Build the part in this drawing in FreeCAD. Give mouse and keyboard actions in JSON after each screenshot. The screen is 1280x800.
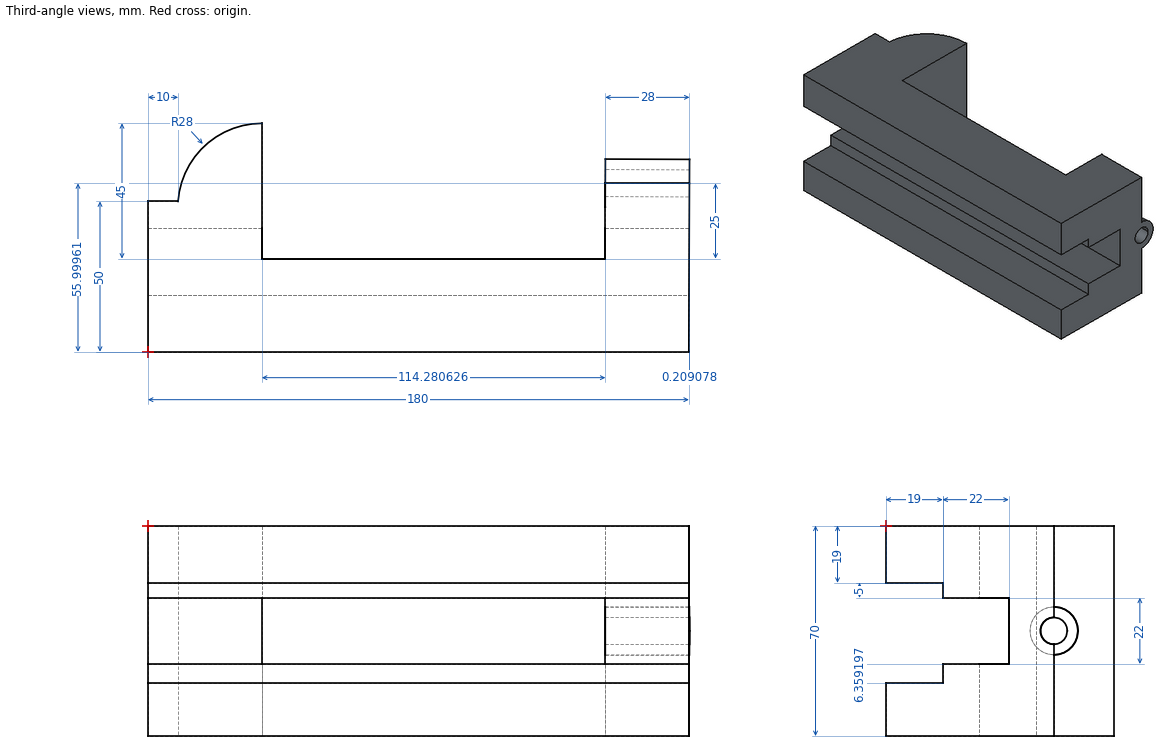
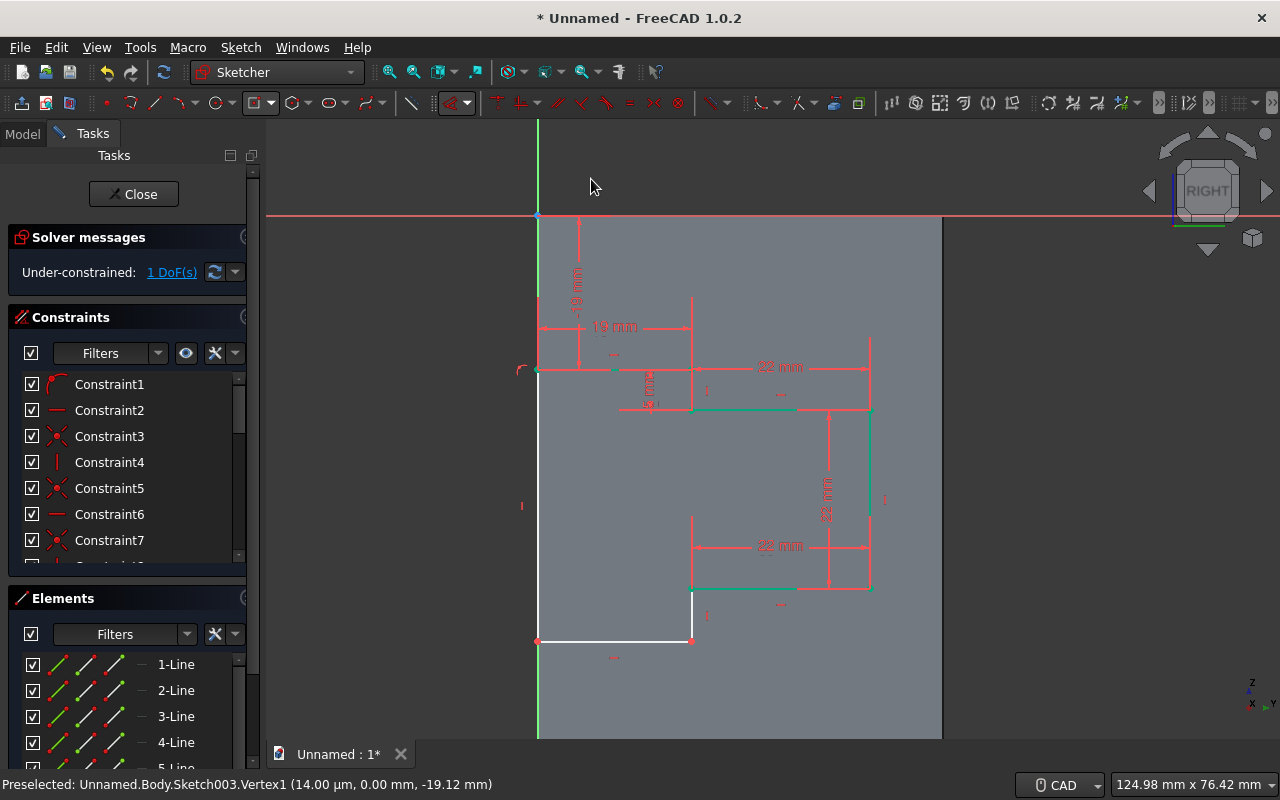
{"action": "left_click", "coordinate": [692, 605]}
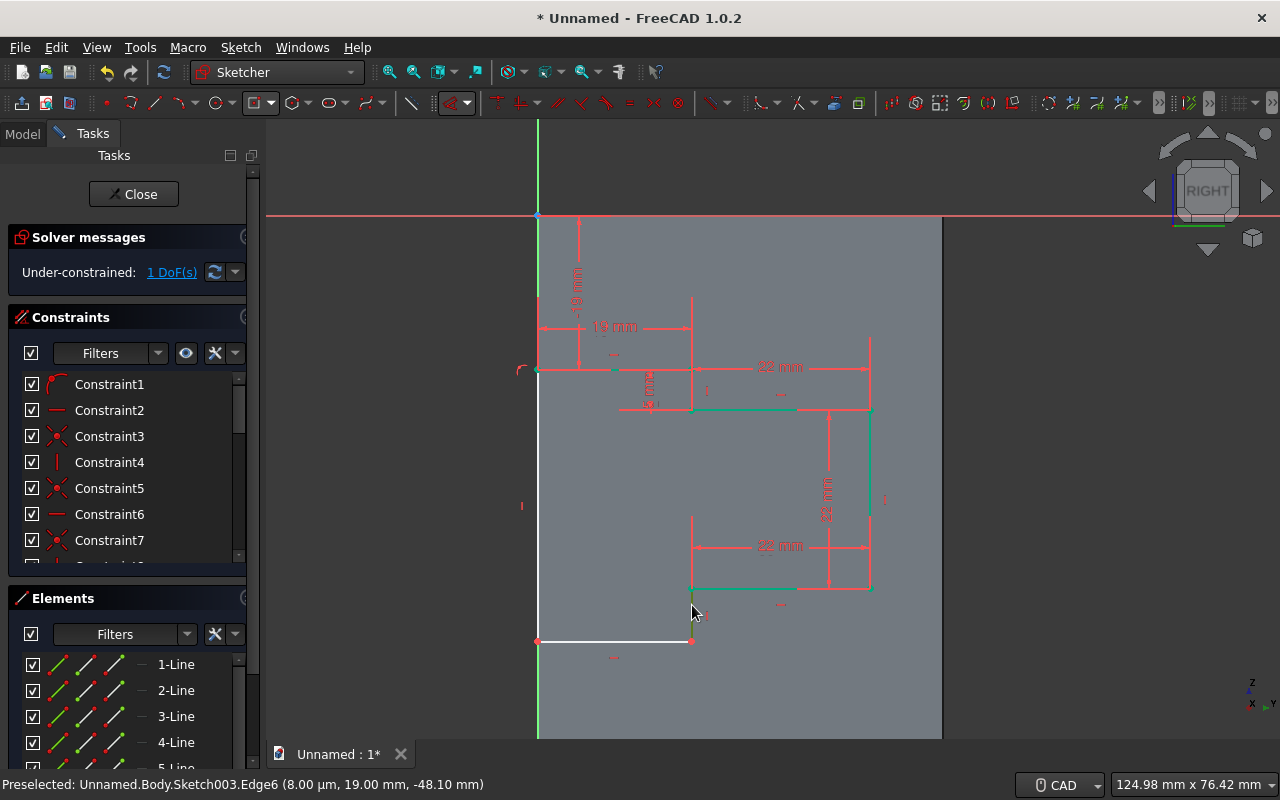
{"action": "left_click", "coordinate": [470, 104]}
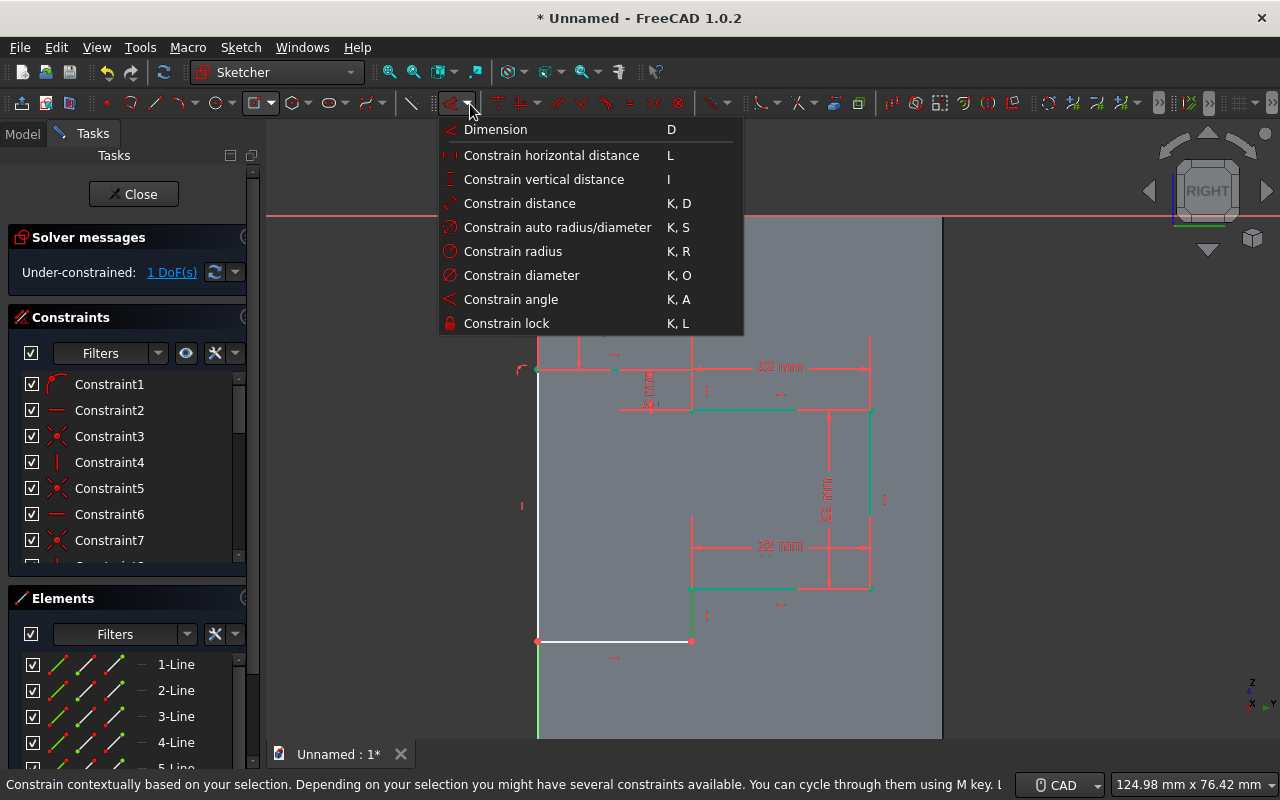
{"action": "left_click", "coordinate": [591, 179]}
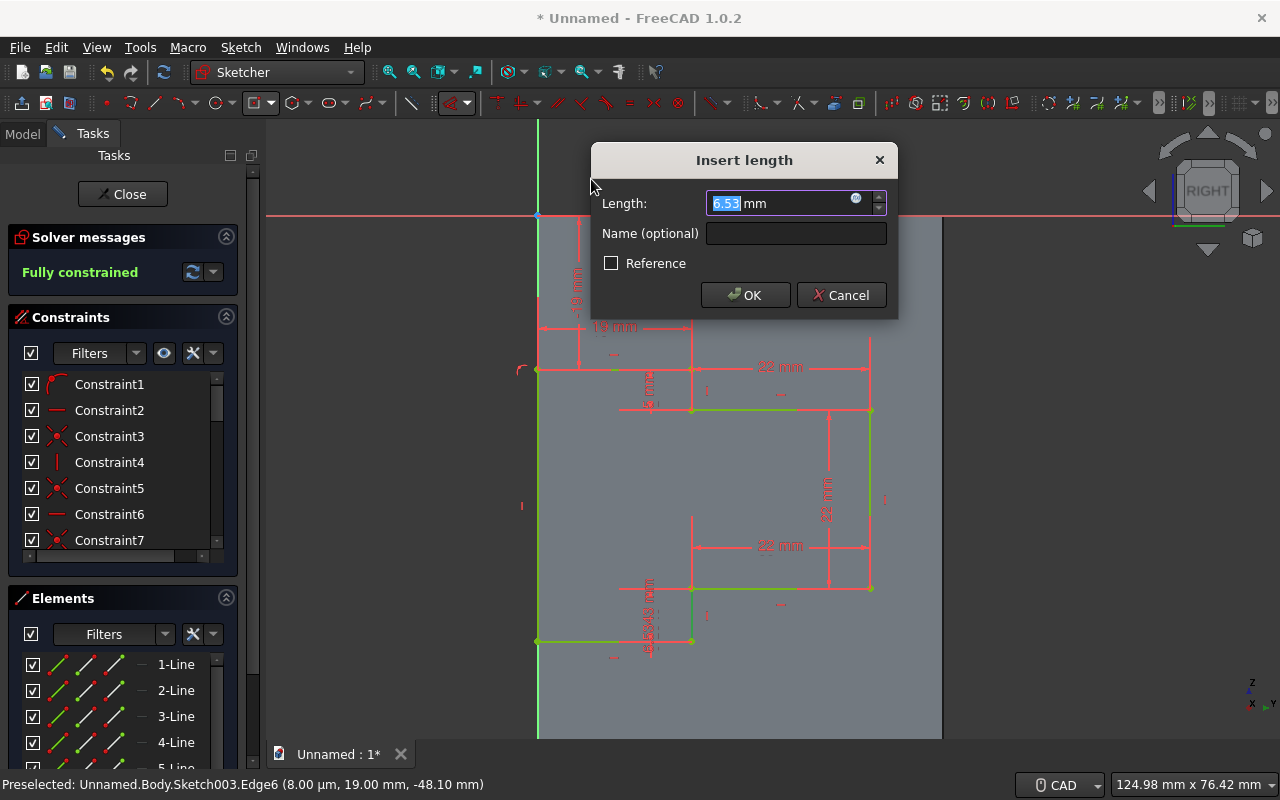
{"action": "type", "text": "6.359197"}
{"action": "key", "text": "Return"}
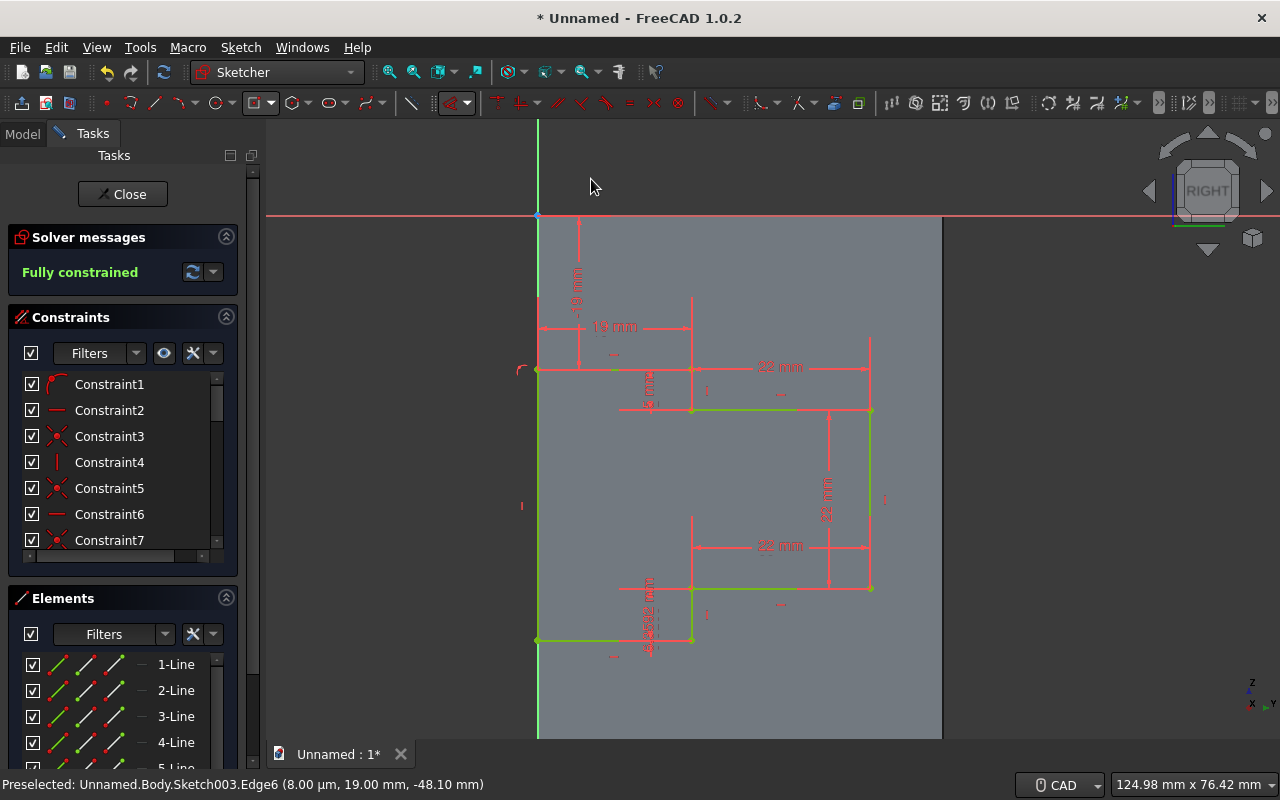
{"action": "left_click", "coordinate": [123, 194]}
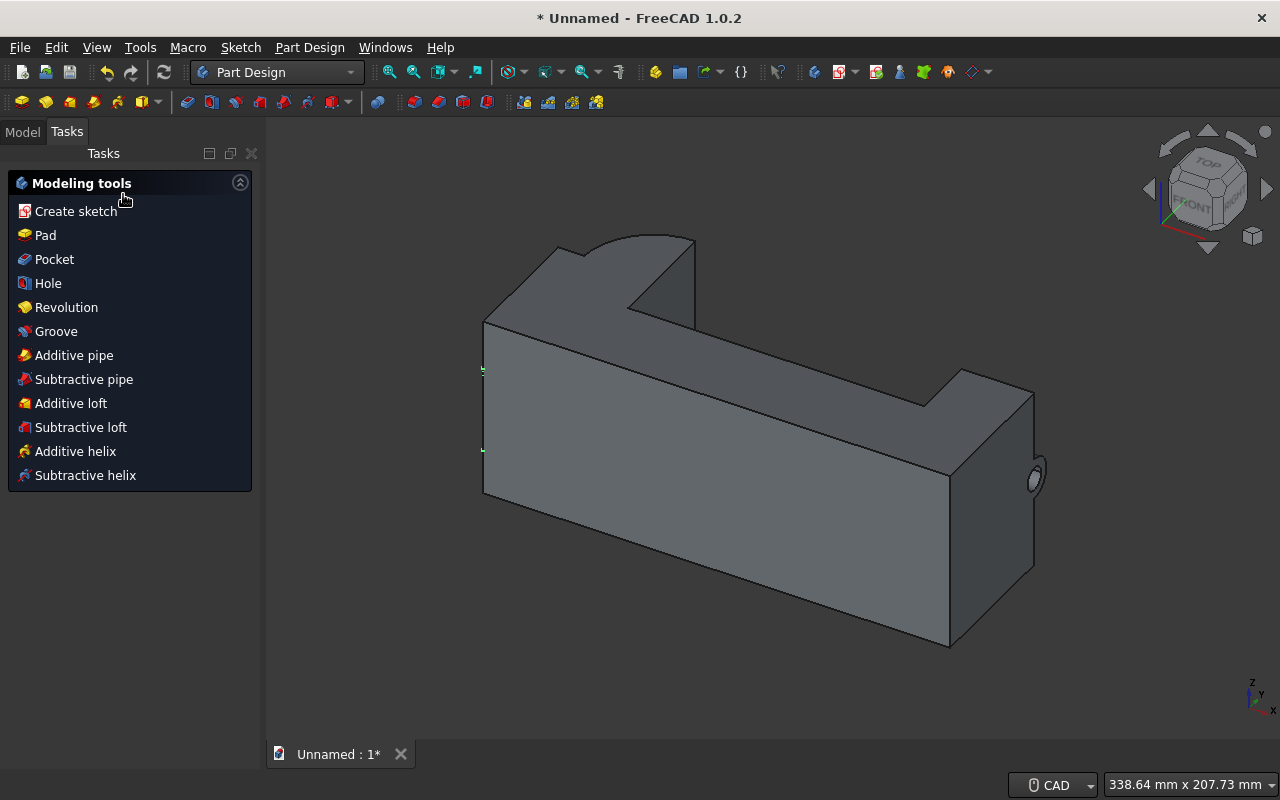
{"action": "left_click", "coordinate": [188, 102]}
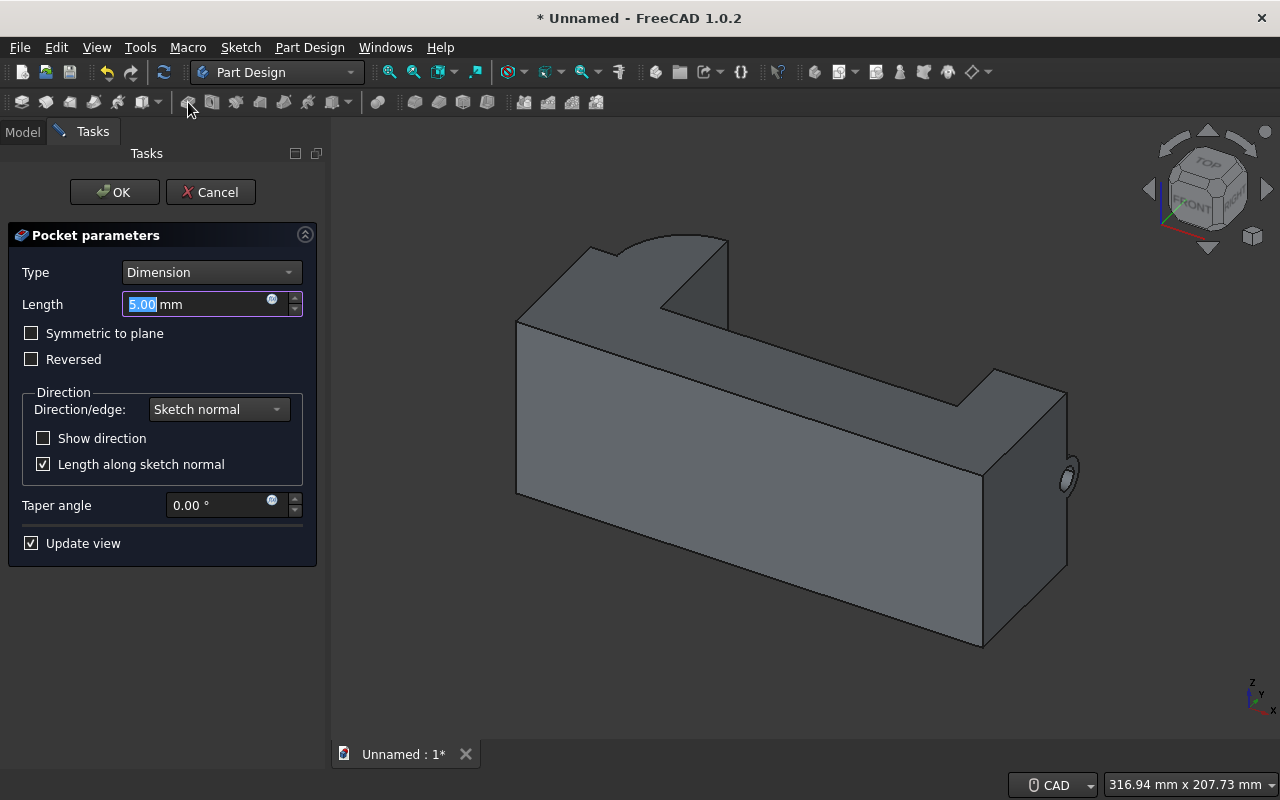
{"action": "left_click", "coordinate": [212, 272]}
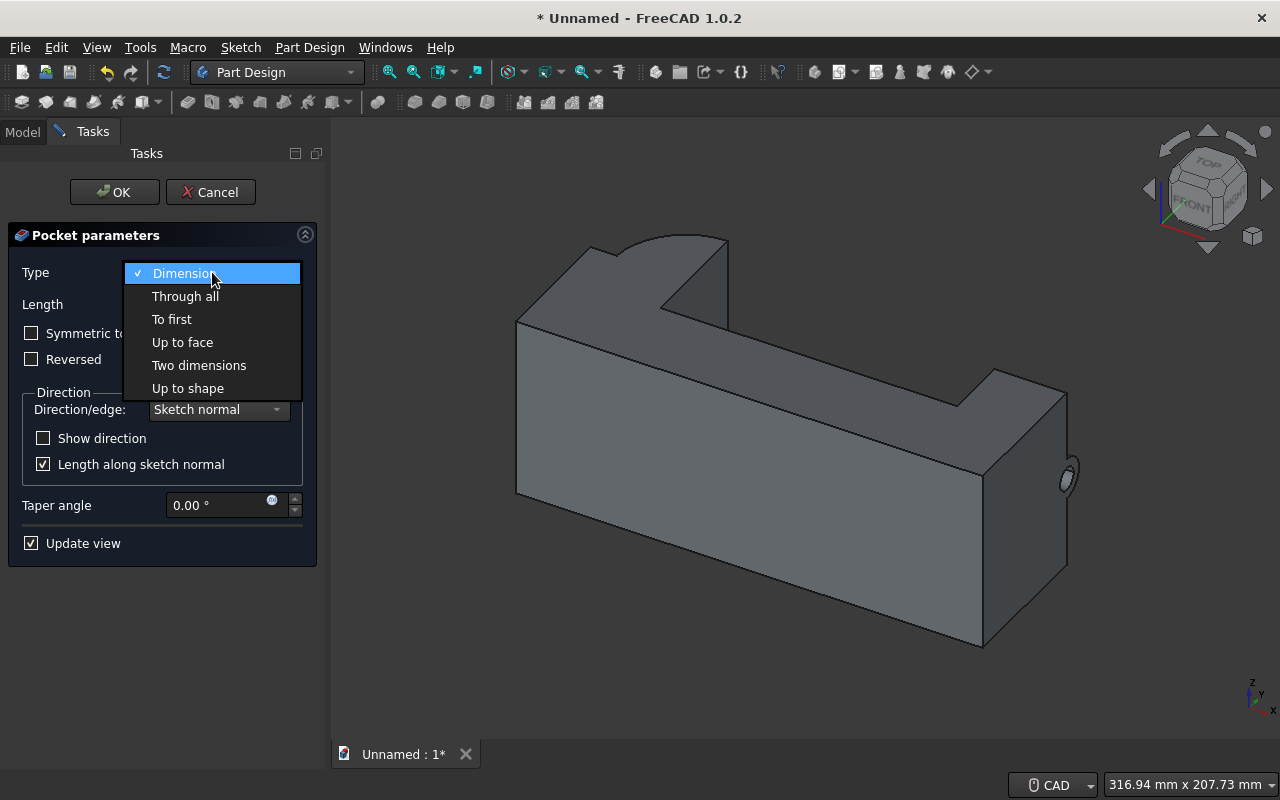
{"action": "left_click", "coordinate": [212, 296]}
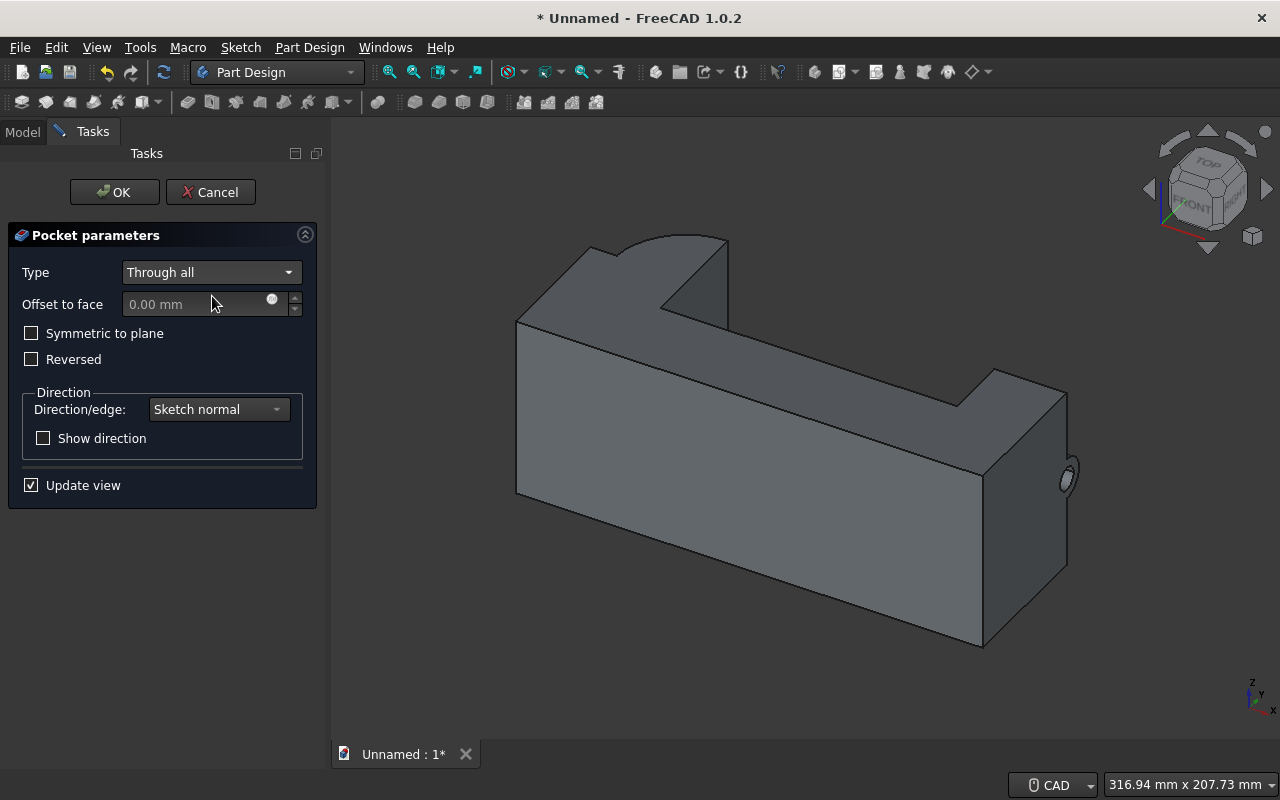
{"action": "left_click", "coordinate": [30, 359]}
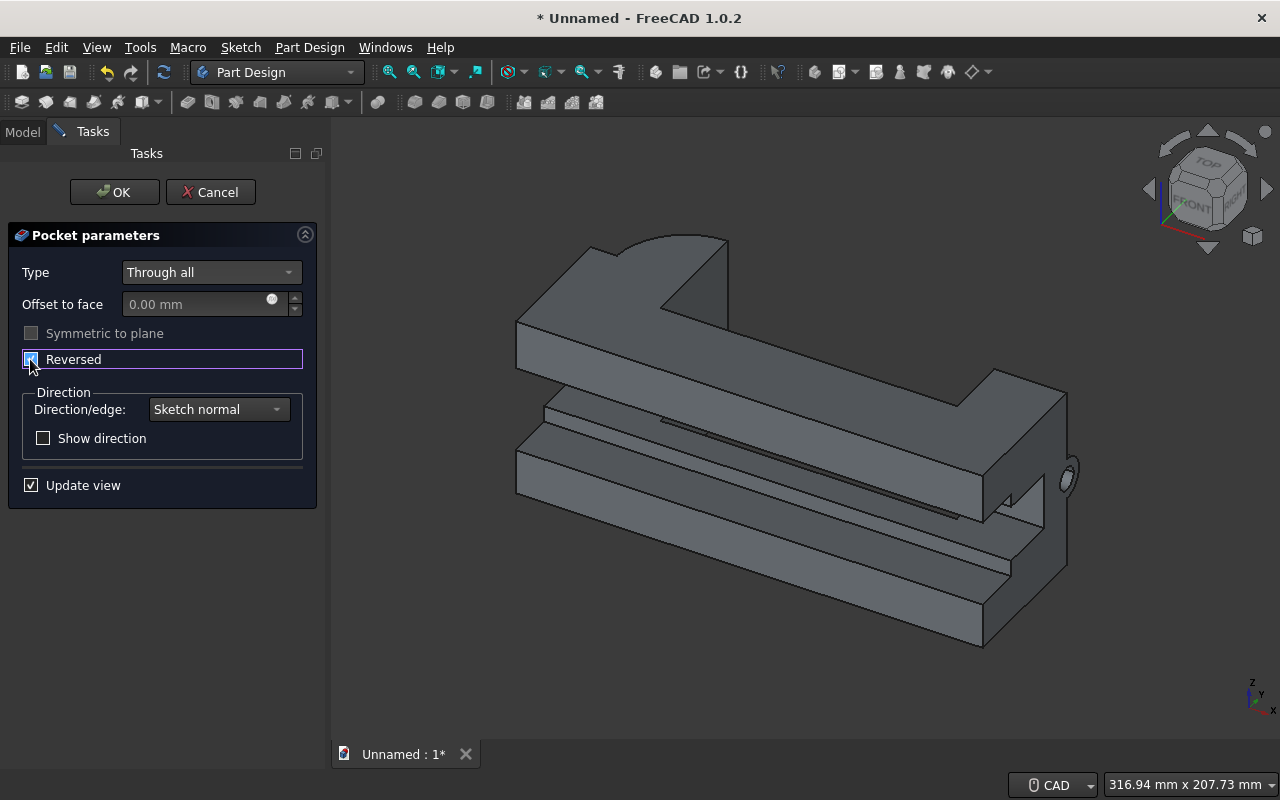
{"action": "left_click", "coordinate": [115, 192]}